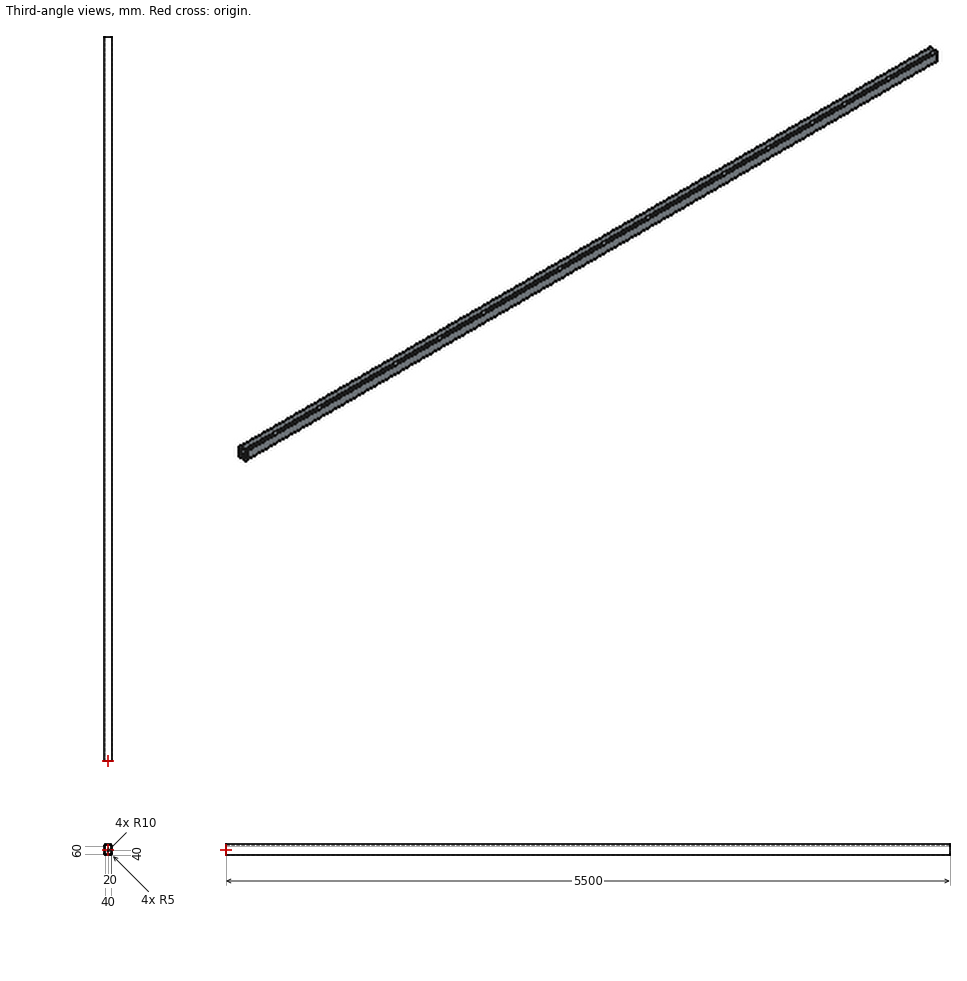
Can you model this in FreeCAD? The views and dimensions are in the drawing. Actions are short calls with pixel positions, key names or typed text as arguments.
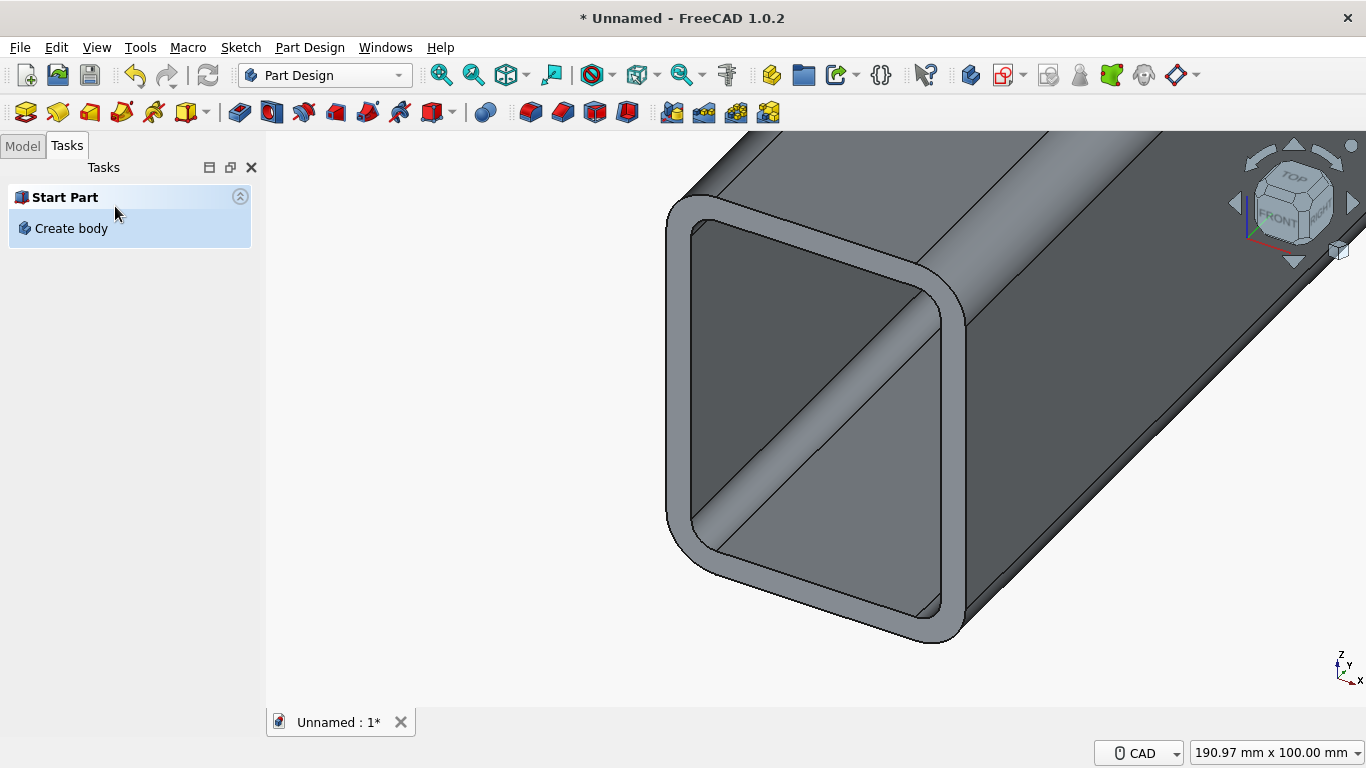
key(0)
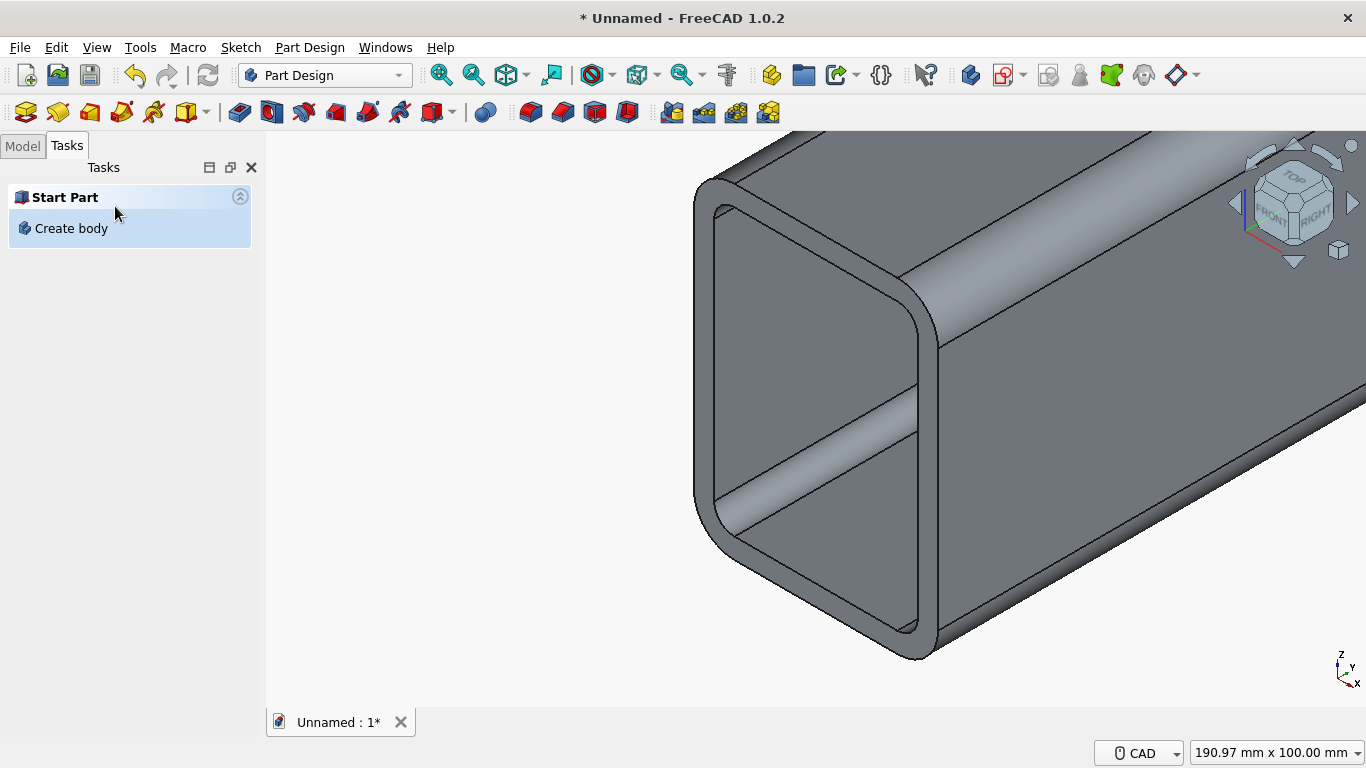
click(442, 76)